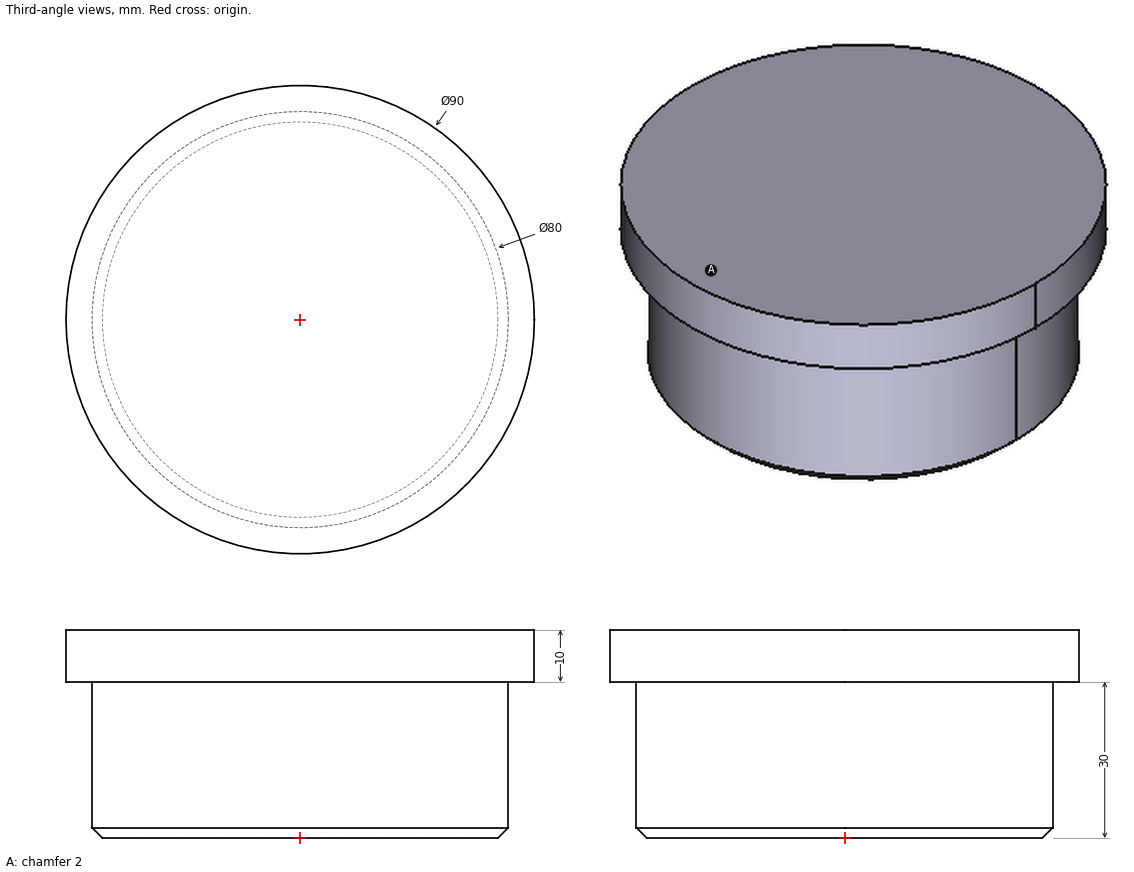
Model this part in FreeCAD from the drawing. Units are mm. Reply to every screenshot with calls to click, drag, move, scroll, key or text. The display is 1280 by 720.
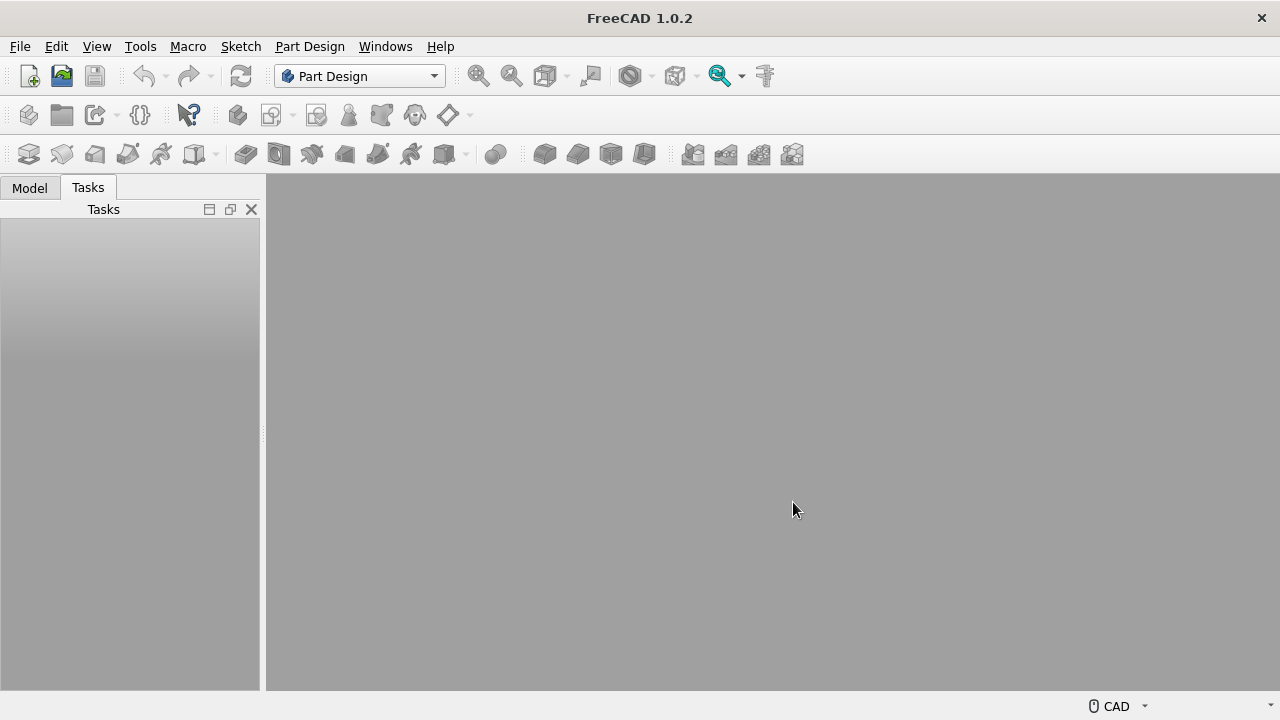
click(29, 76)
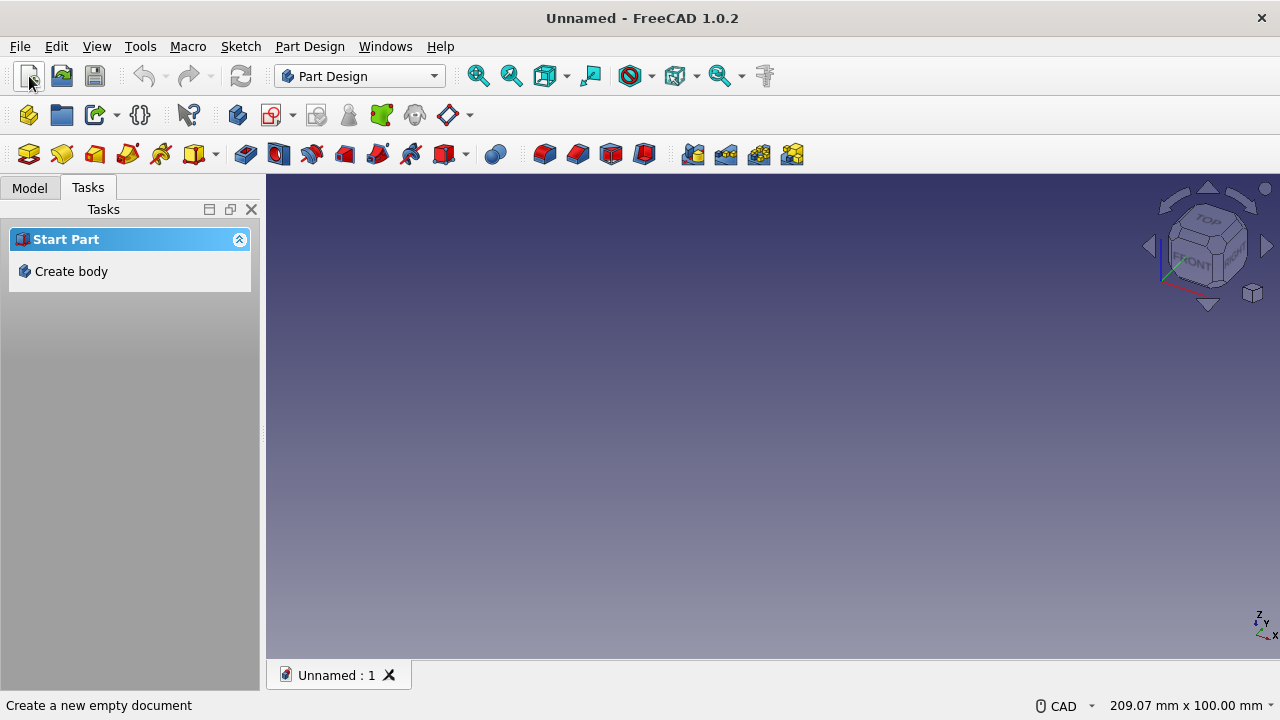
click(270, 116)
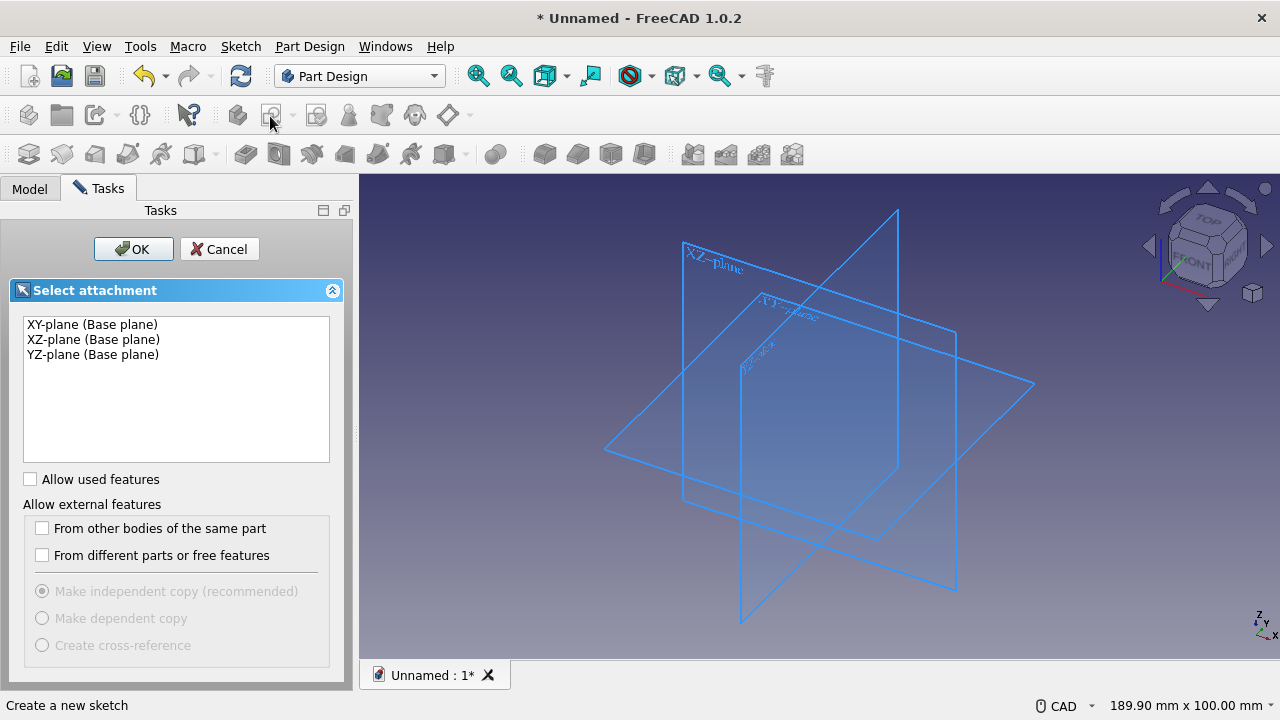
click(84, 324)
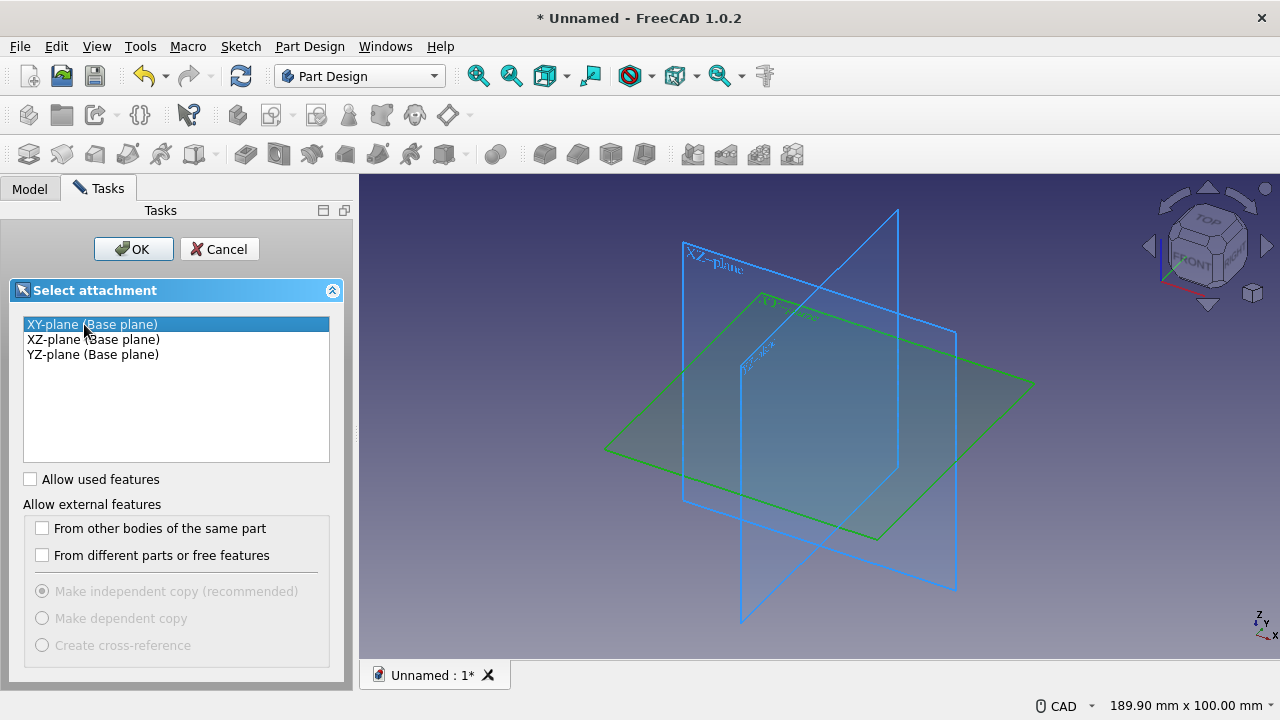
click(134, 249)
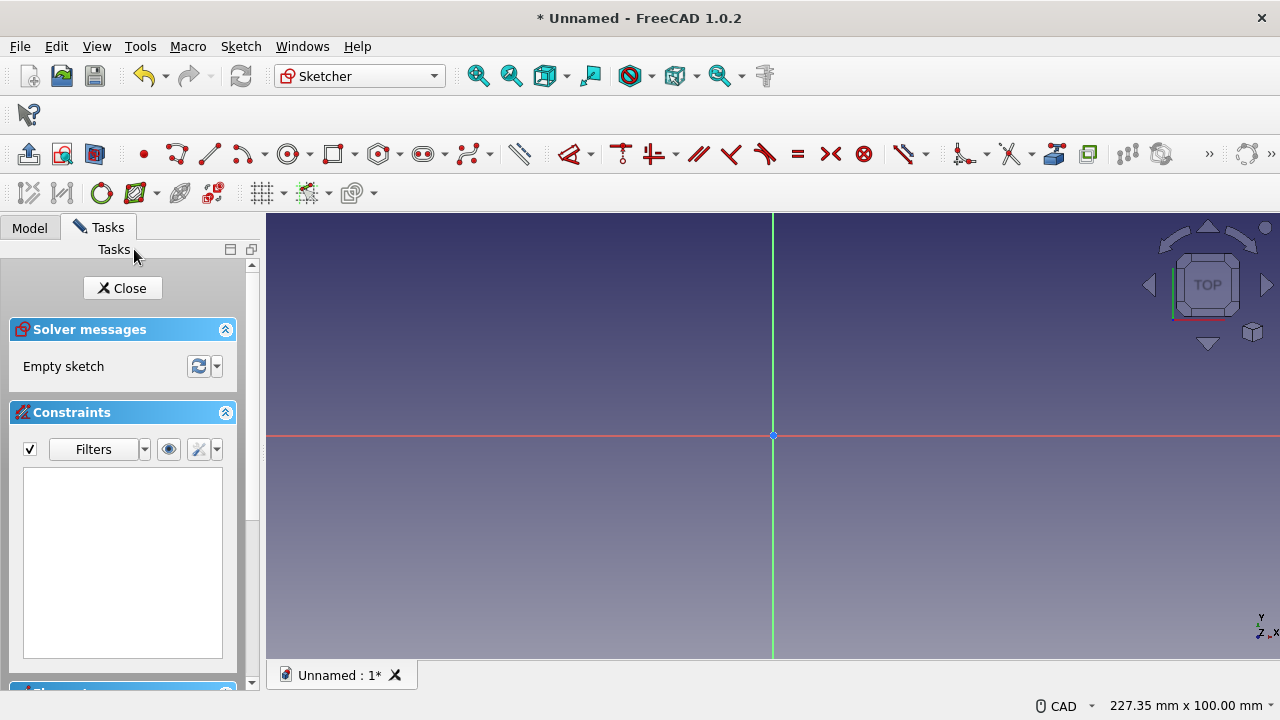
scroll(395, 436, down, 1)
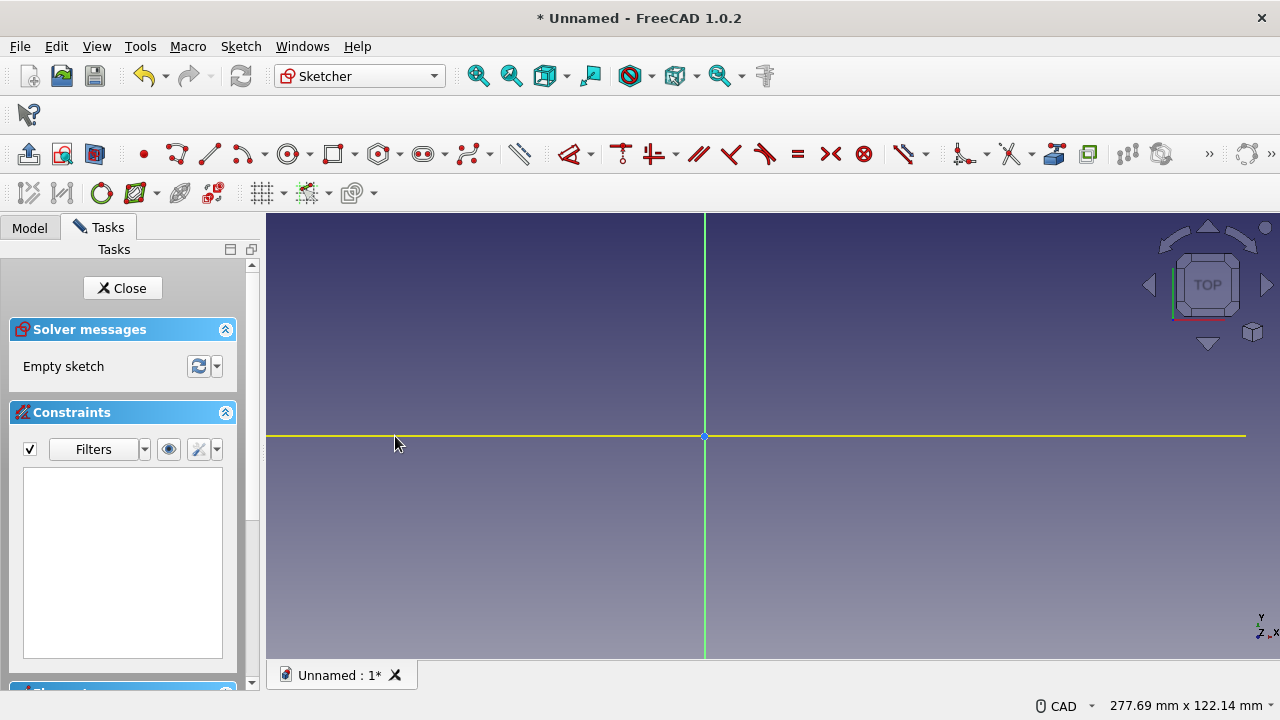
click(288, 154)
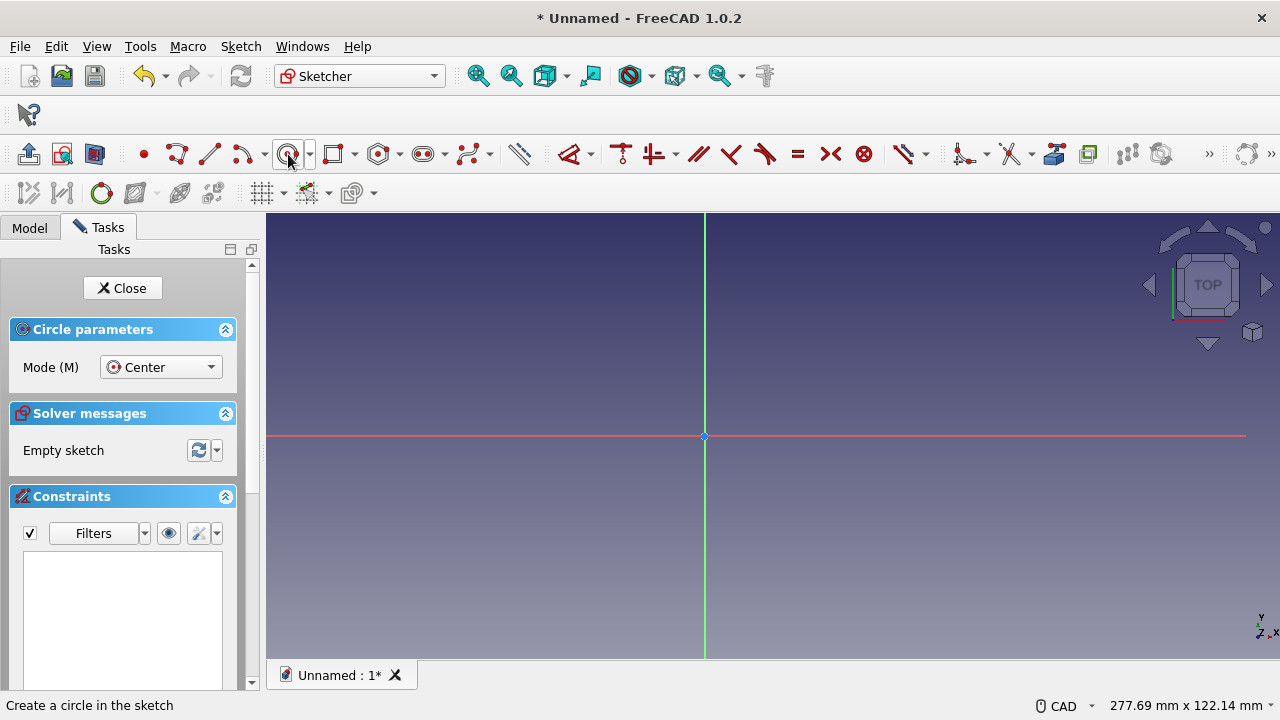
click(705, 436)
move(808, 333)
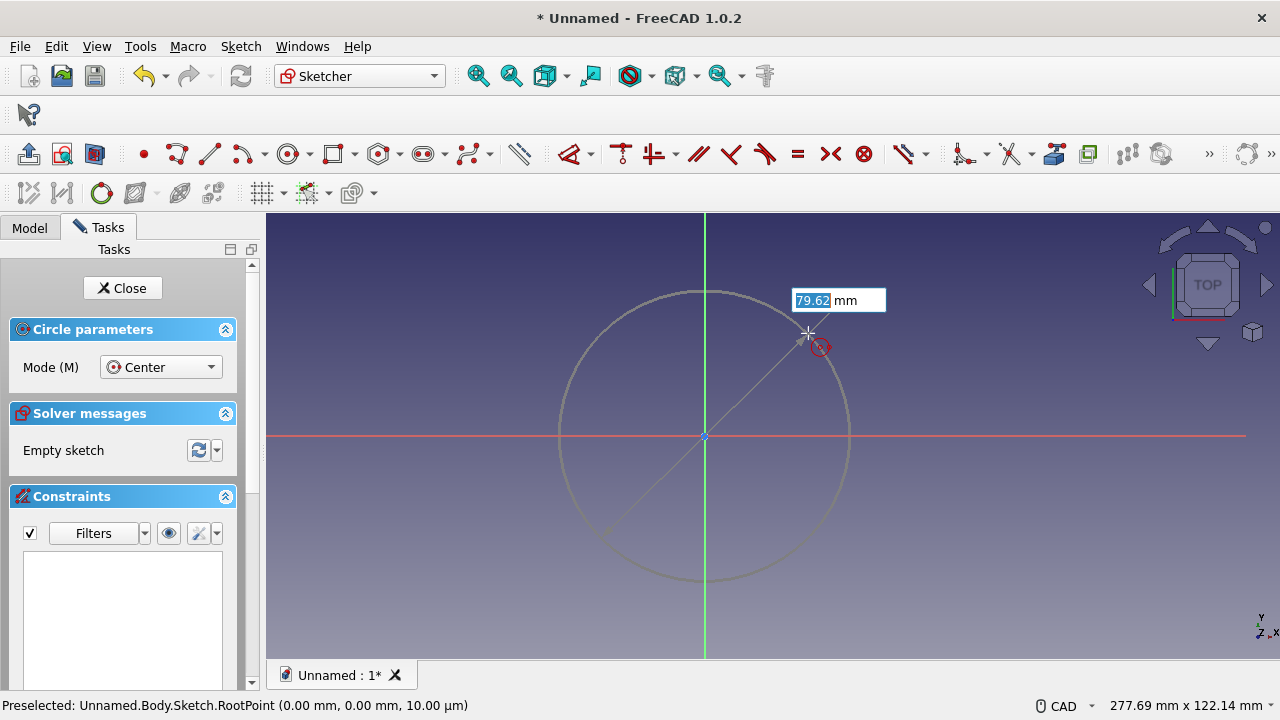
text(80)
key(Return)
key(Escape)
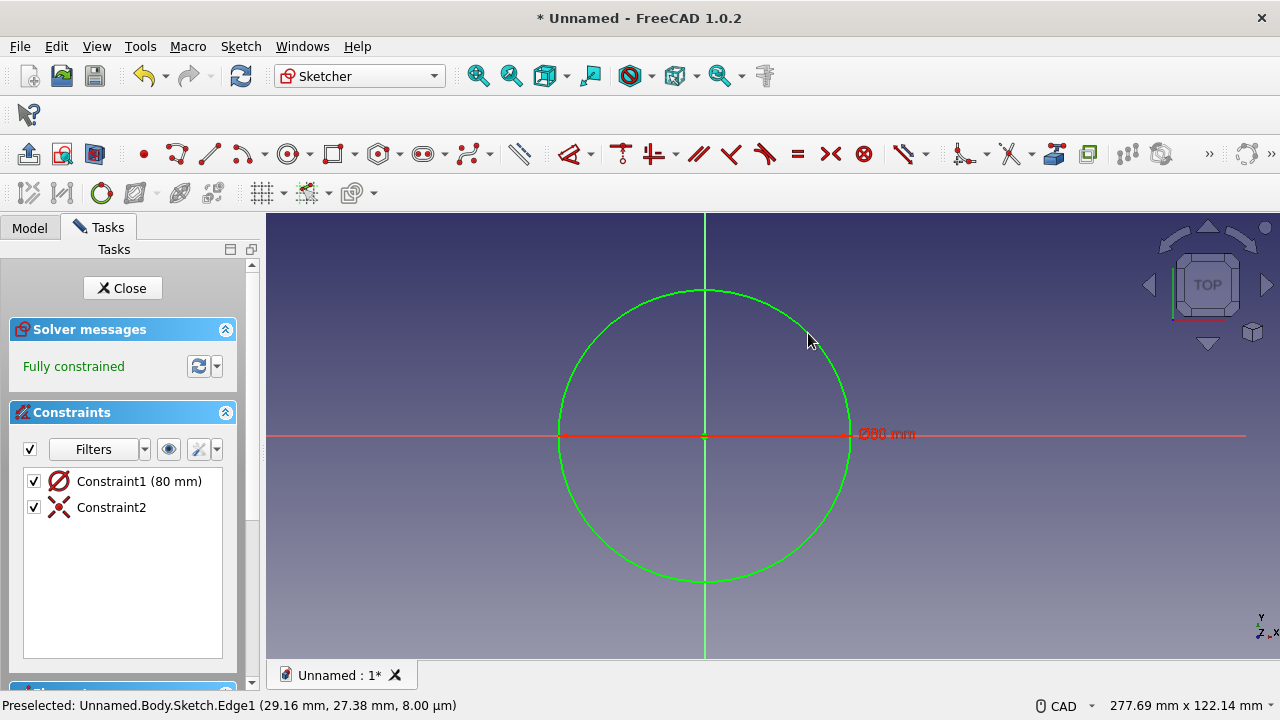
click(123, 288)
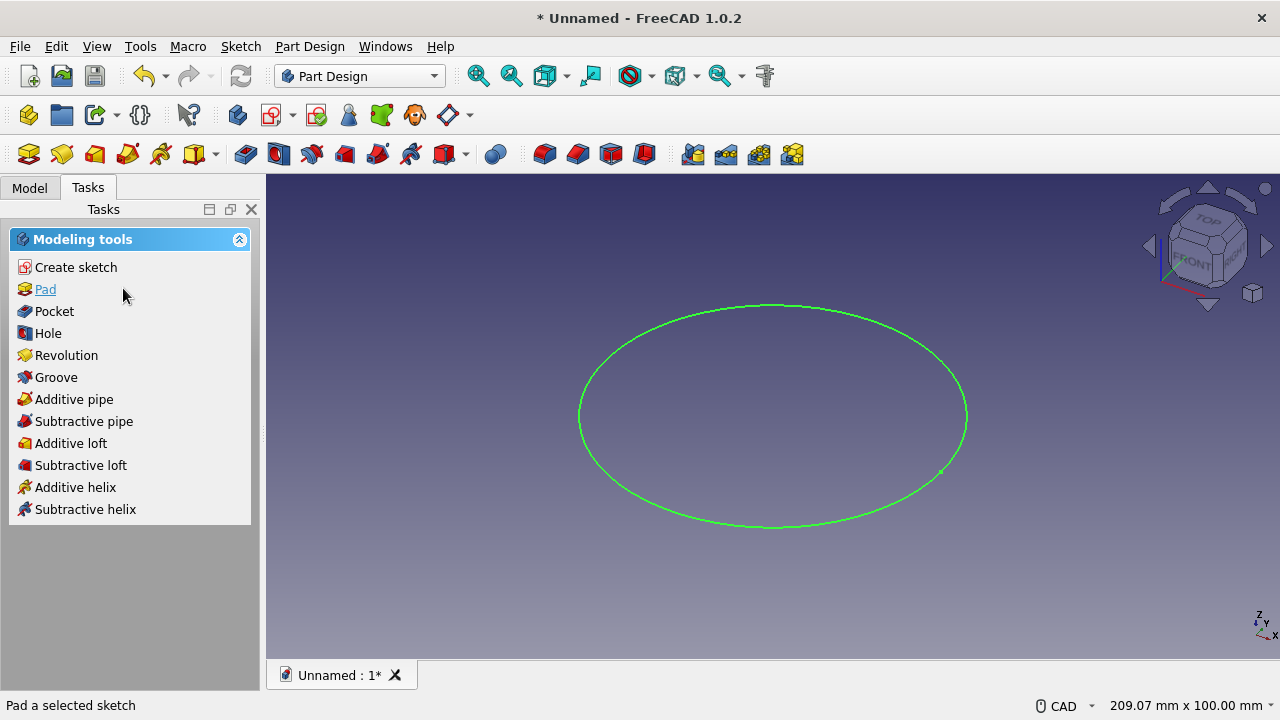
click(29, 154)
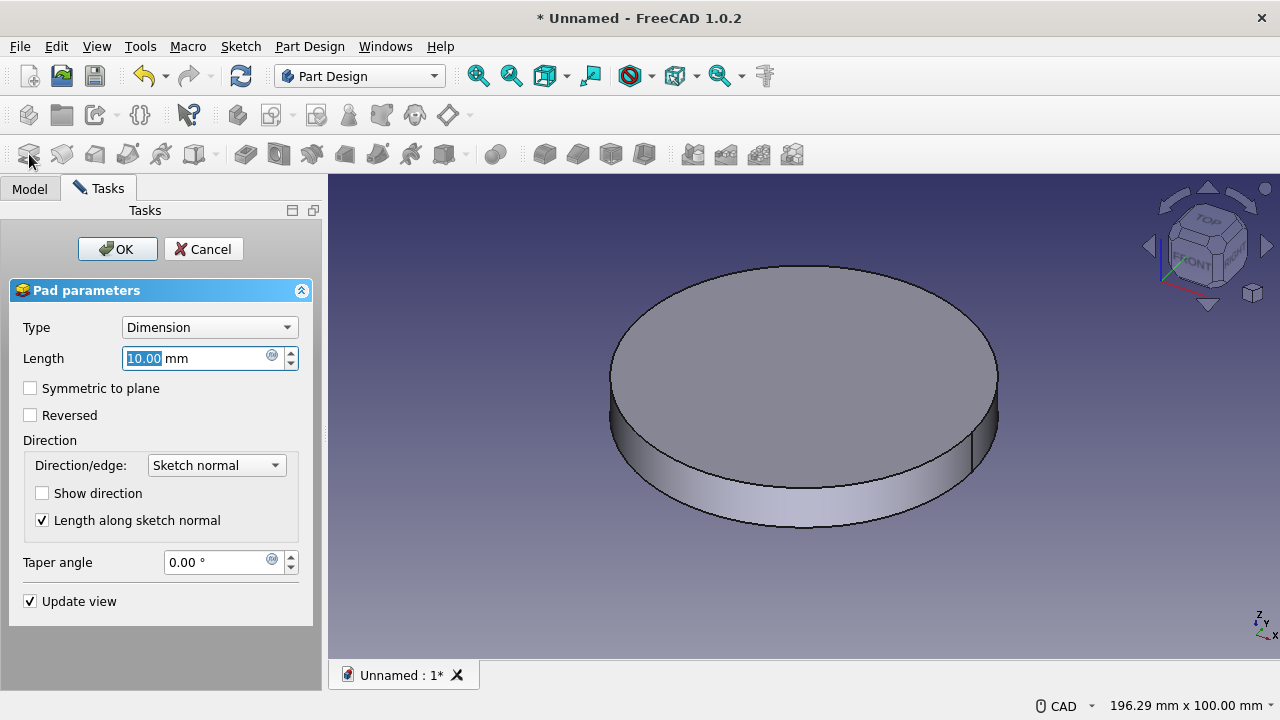
text(30)
key(Tab)